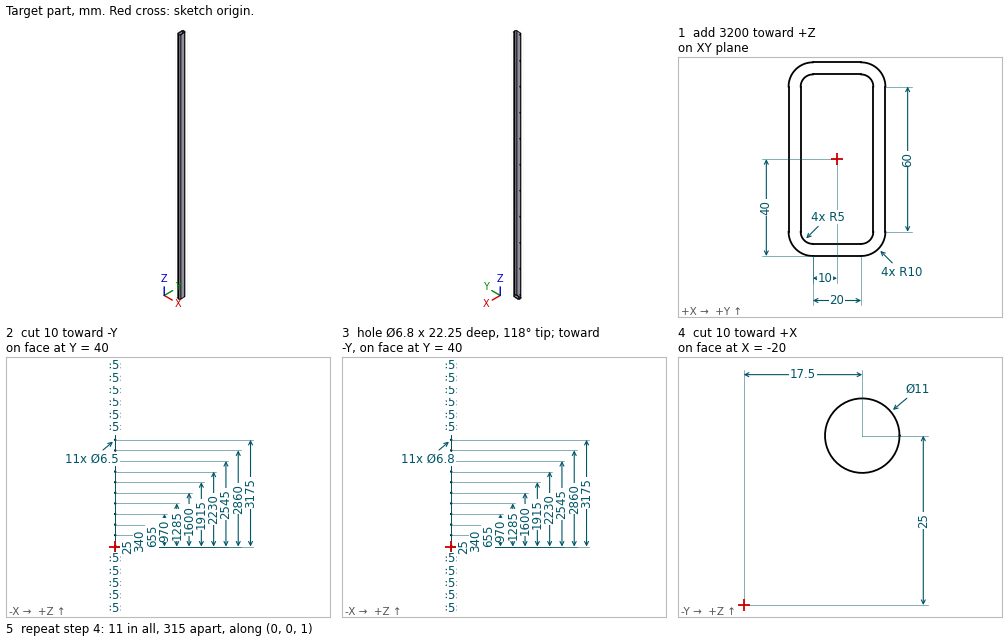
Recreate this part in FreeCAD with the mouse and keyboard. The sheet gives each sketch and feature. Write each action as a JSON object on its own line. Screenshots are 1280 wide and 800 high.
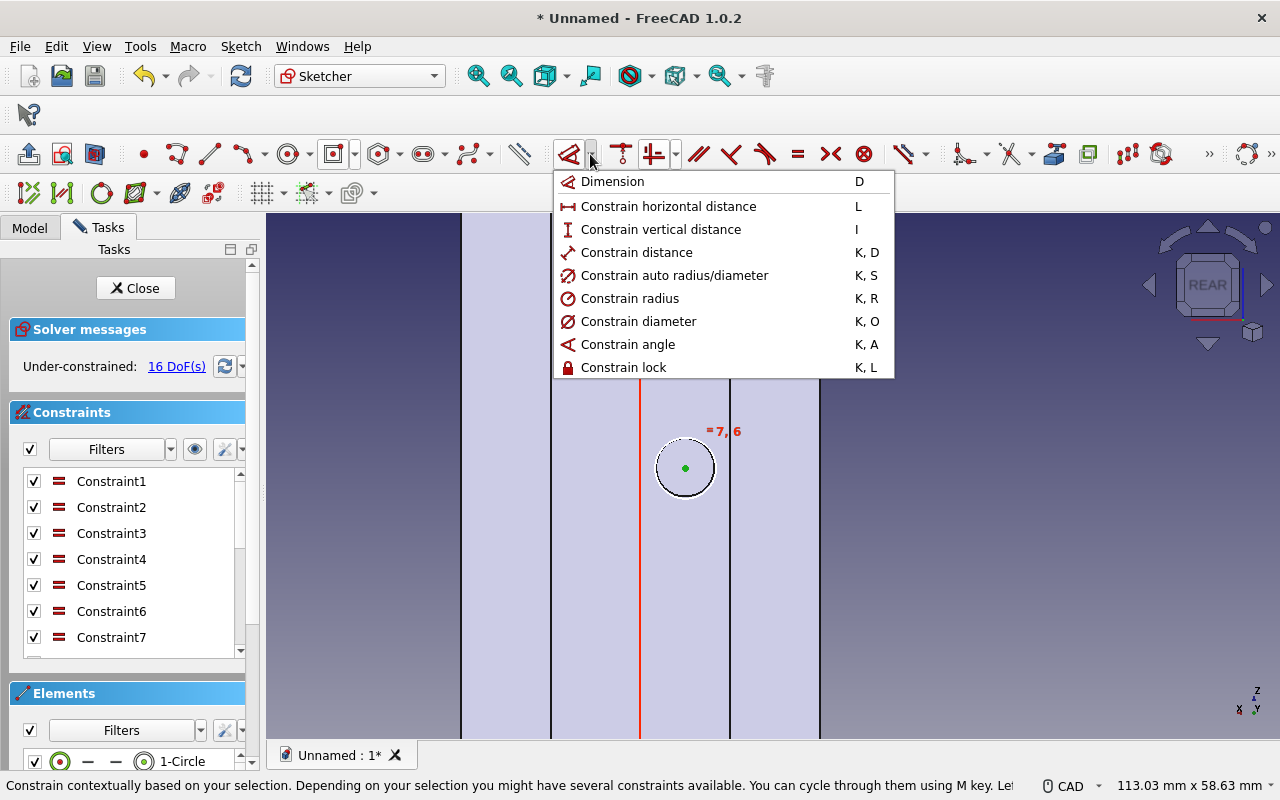
{"action": "left_click", "coordinate": [724, 206]}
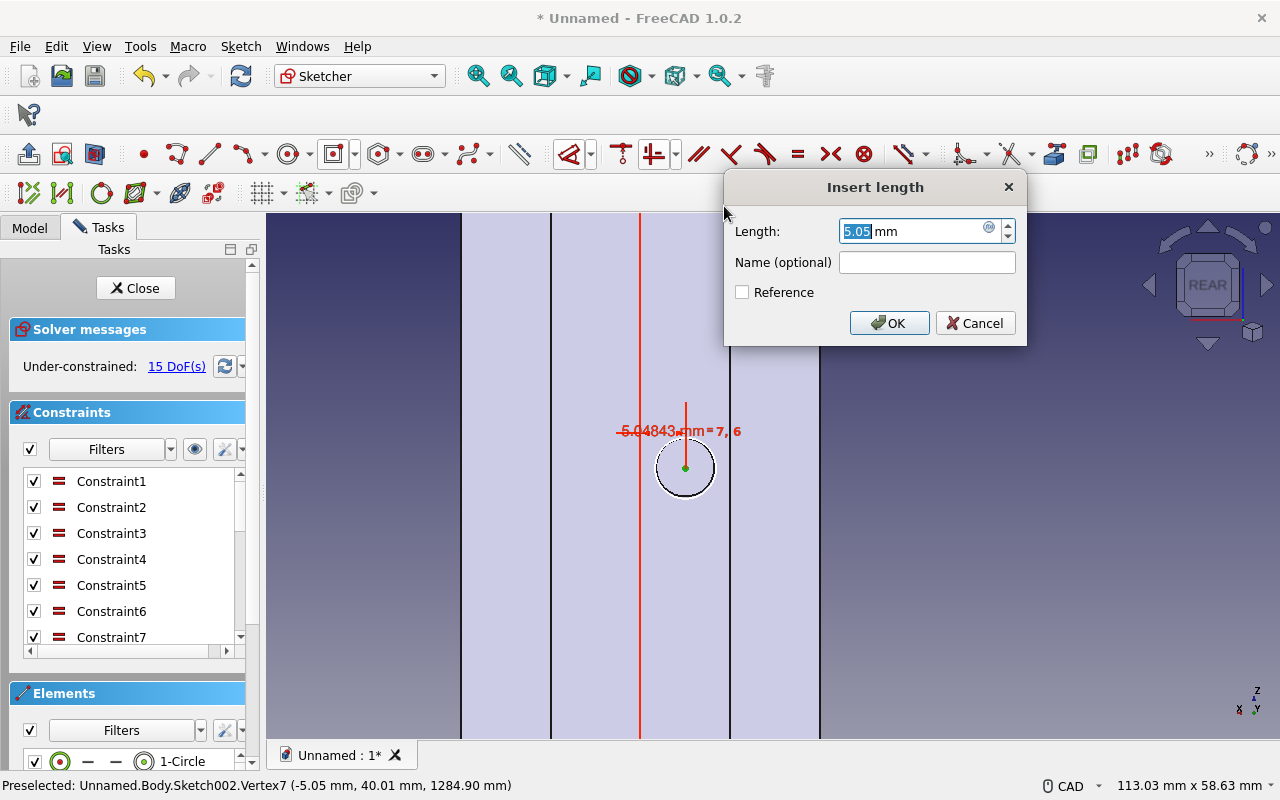
{"action": "type", "text": "5"}
{"action": "key", "text": "Return"}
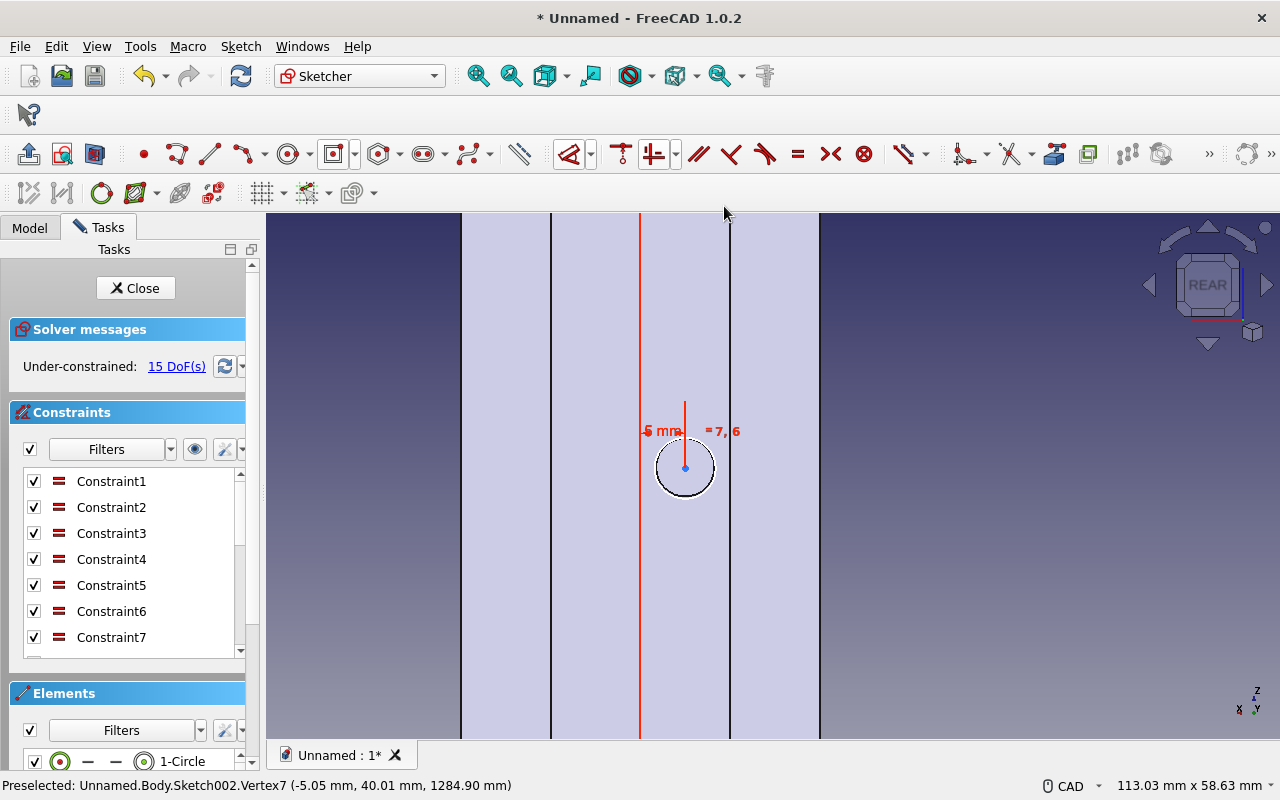
{"action": "scroll", "coordinate": [704, 476], "scroll_direction": "down", "scroll_amount": 15}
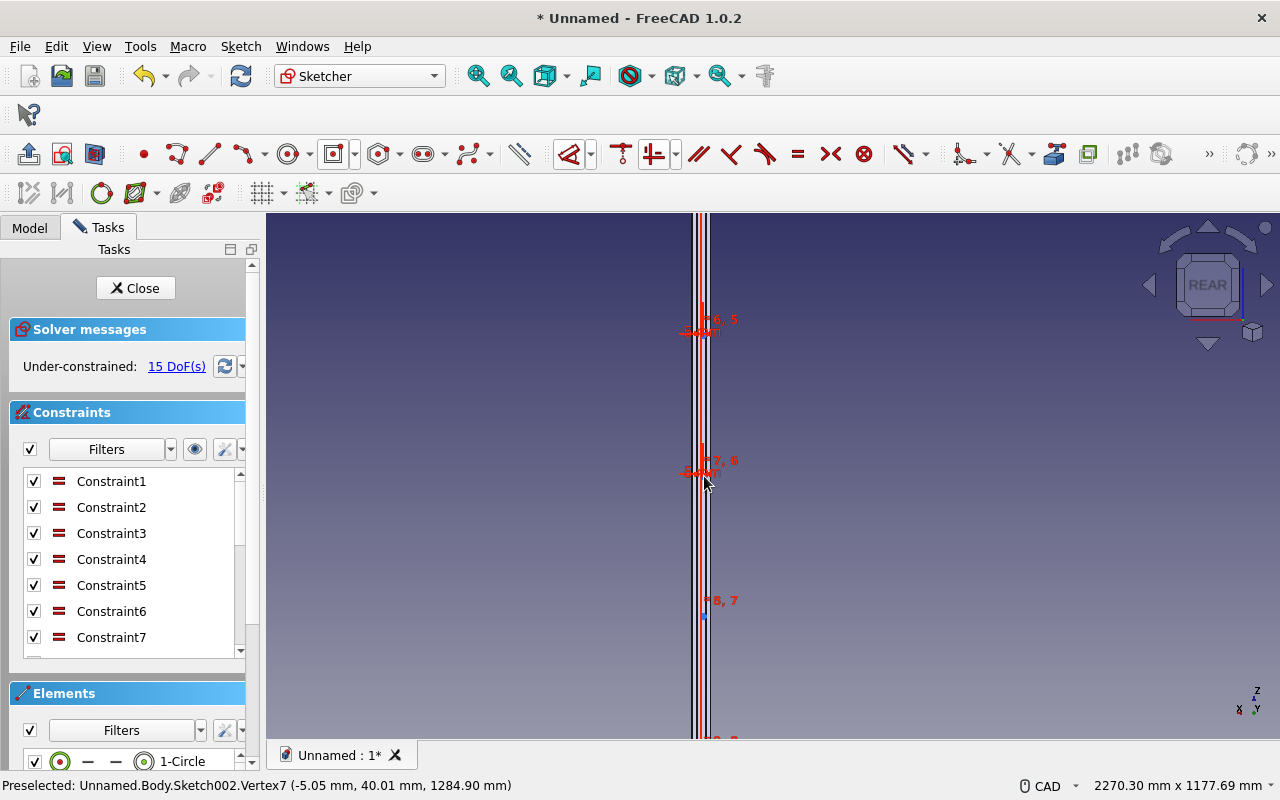
{"action": "scroll", "coordinate": [705, 520], "scroll_direction": "down", "scroll_amount": 7}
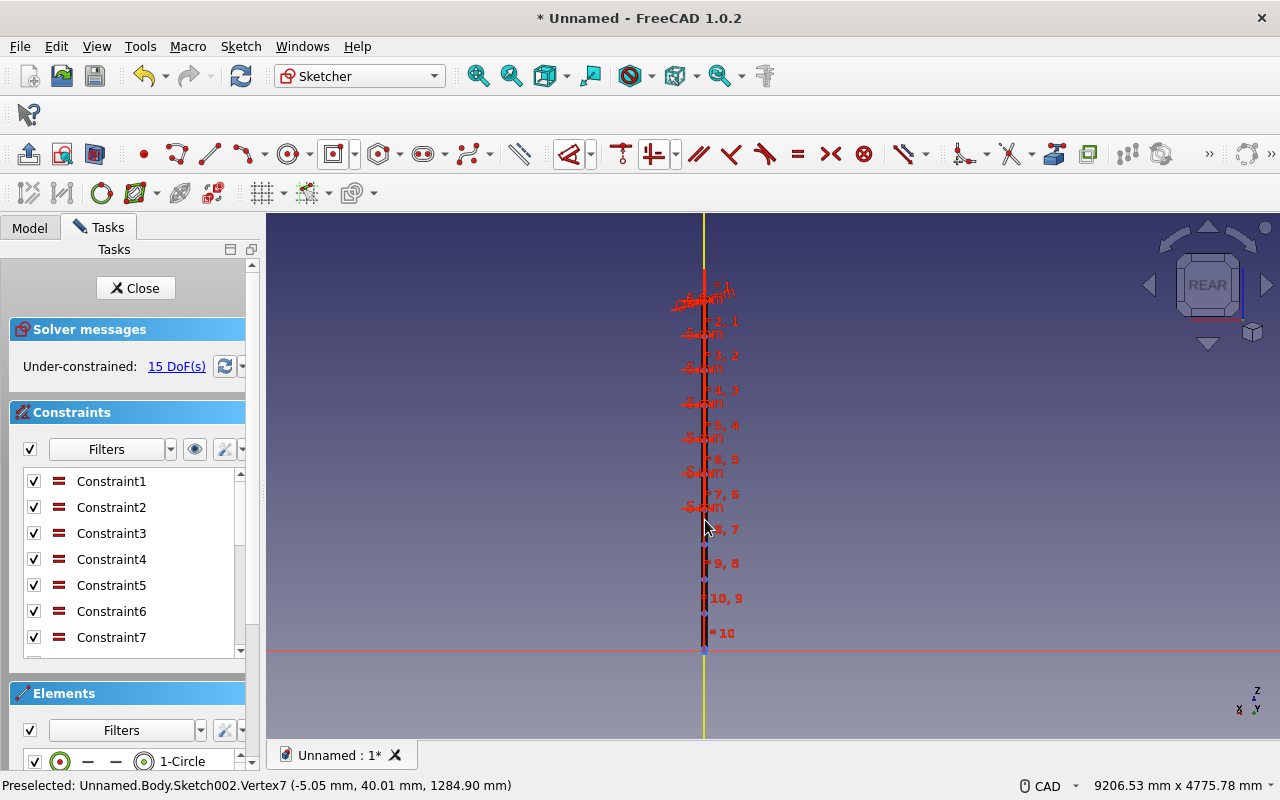
{"action": "scroll", "coordinate": [705, 544], "scroll_direction": "up", "scroll_amount": 22}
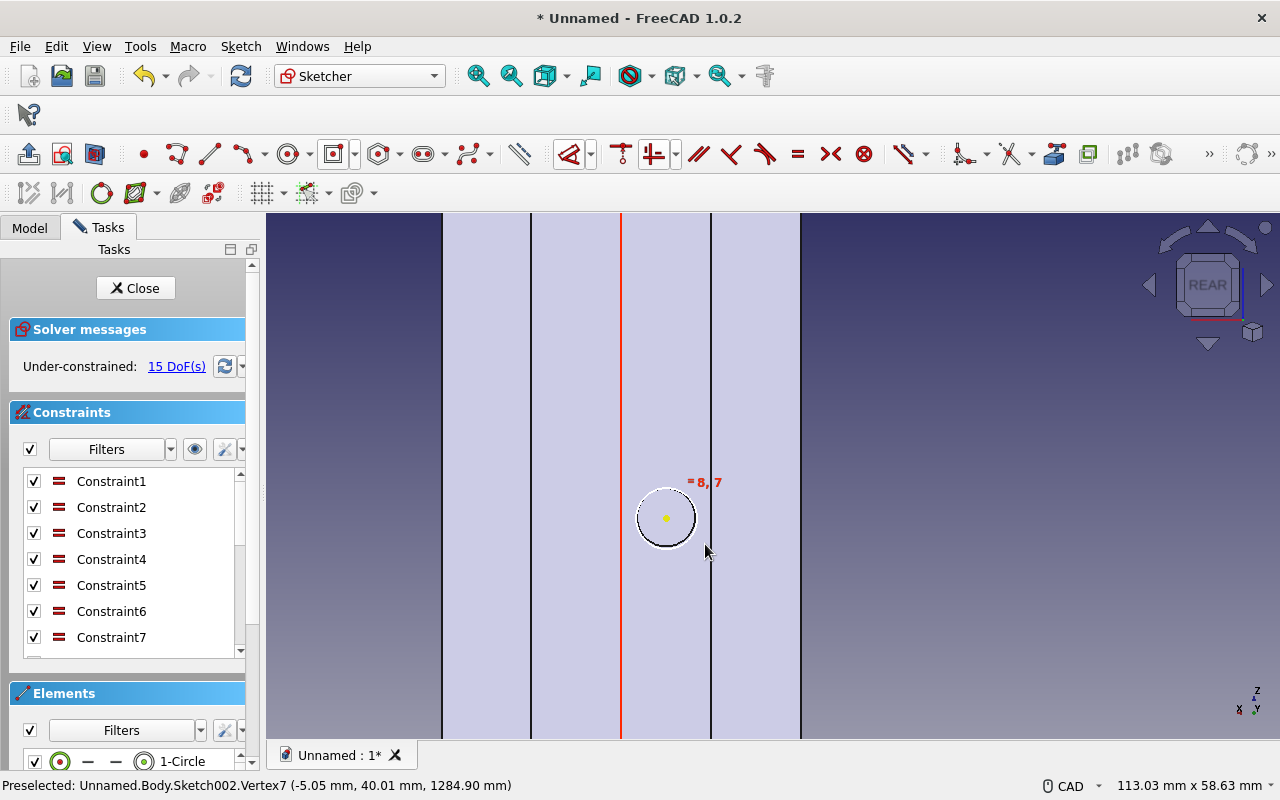
{"action": "left_click", "coordinate": [667, 519]}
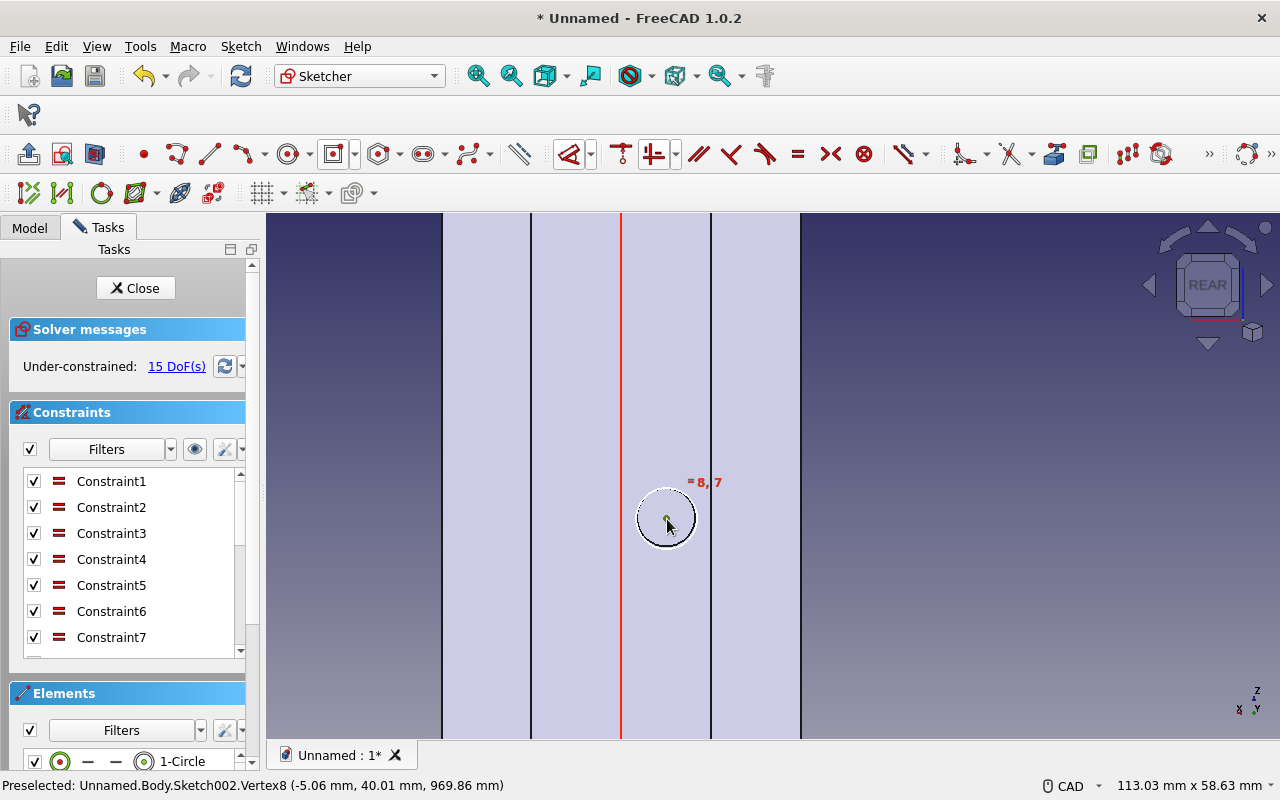
{"action": "key", "text": "l"}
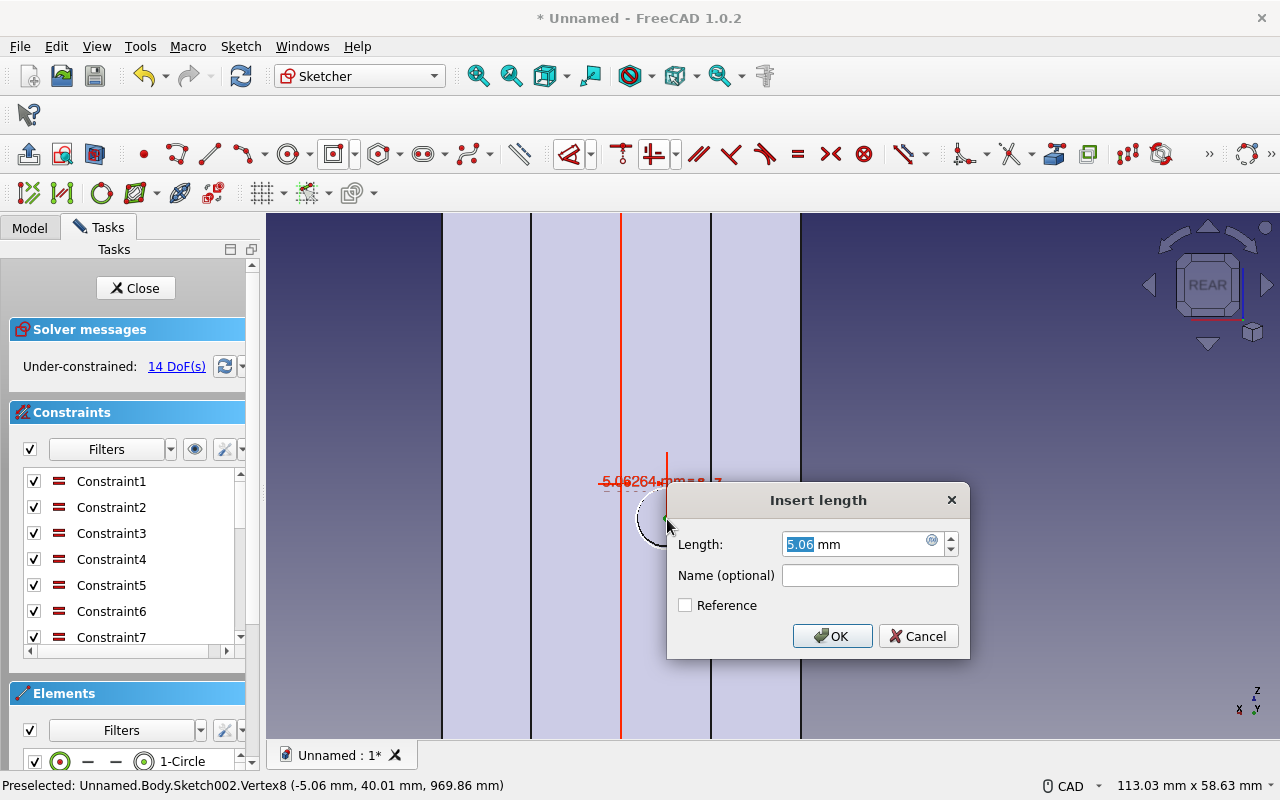
{"action": "type", "text": "5"}
{"action": "key", "text": "Return"}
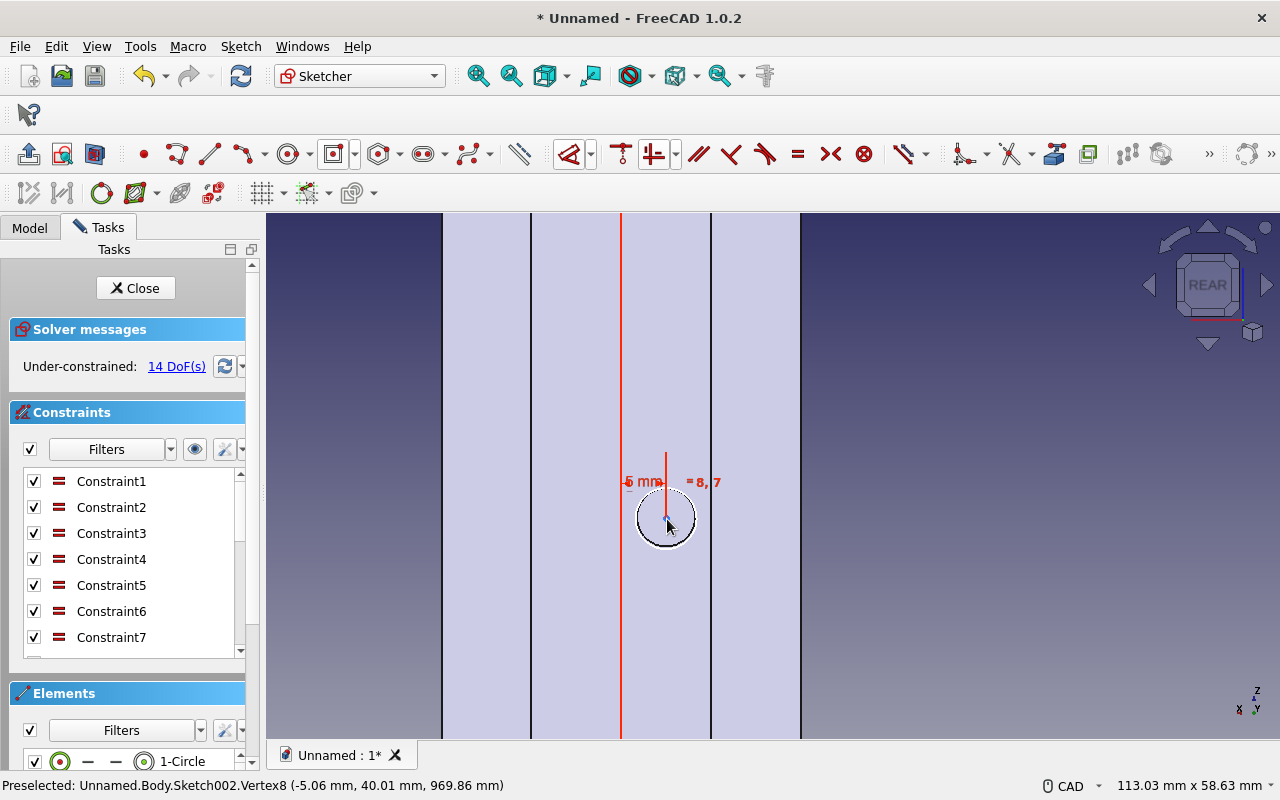
{"action": "scroll", "coordinate": [704, 476], "scroll_direction": "down", "scroll_amount": 15}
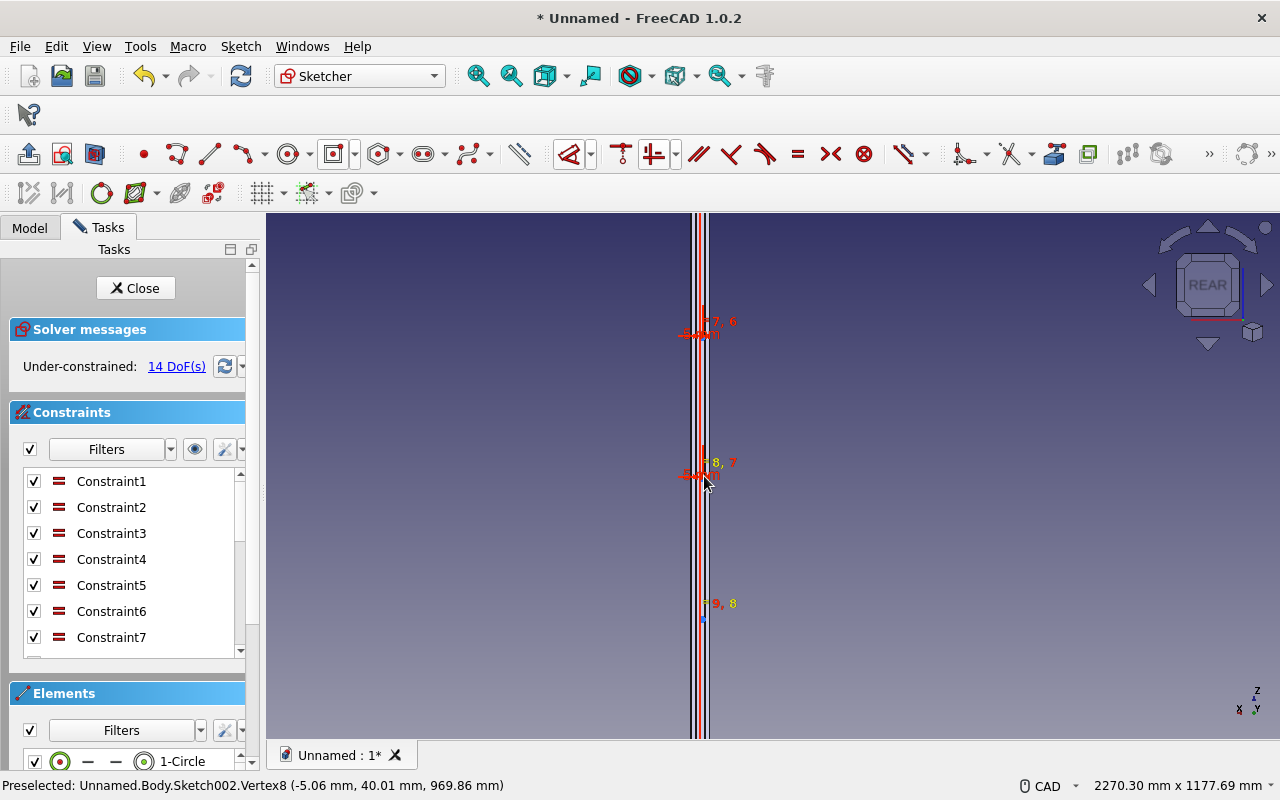
{"action": "scroll", "coordinate": [705, 566], "scroll_direction": "down", "scroll_amount": 7}